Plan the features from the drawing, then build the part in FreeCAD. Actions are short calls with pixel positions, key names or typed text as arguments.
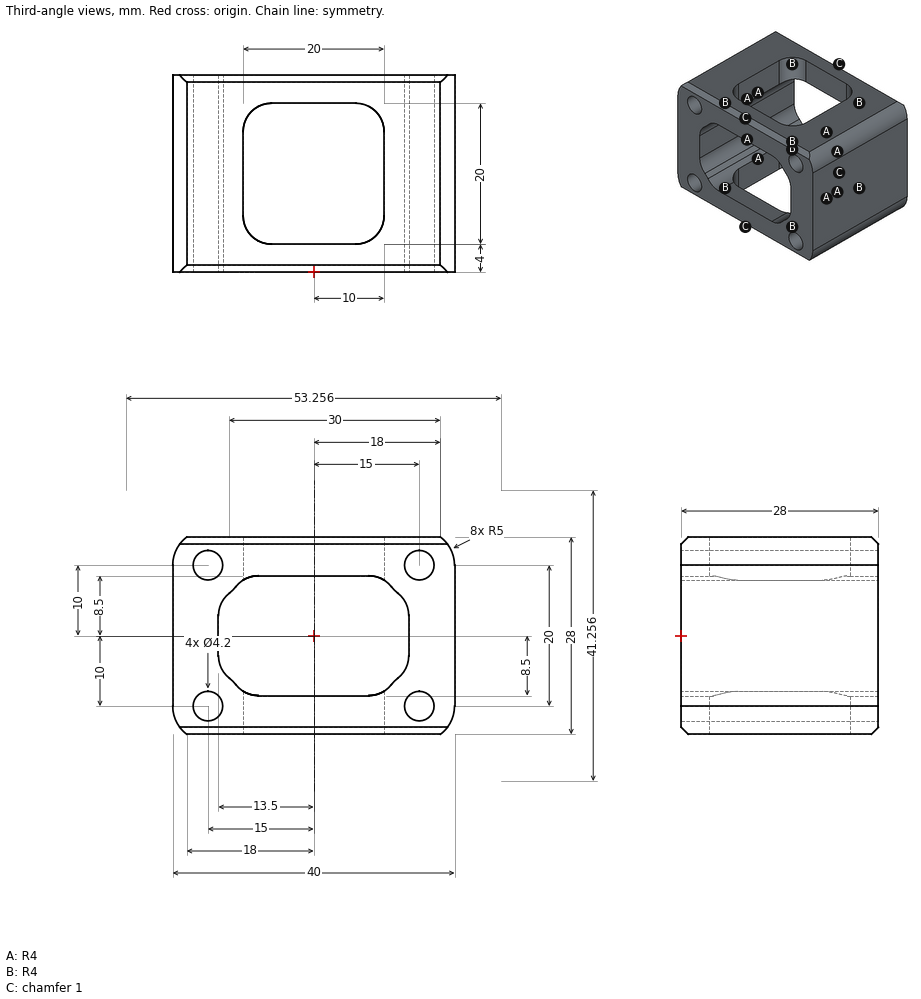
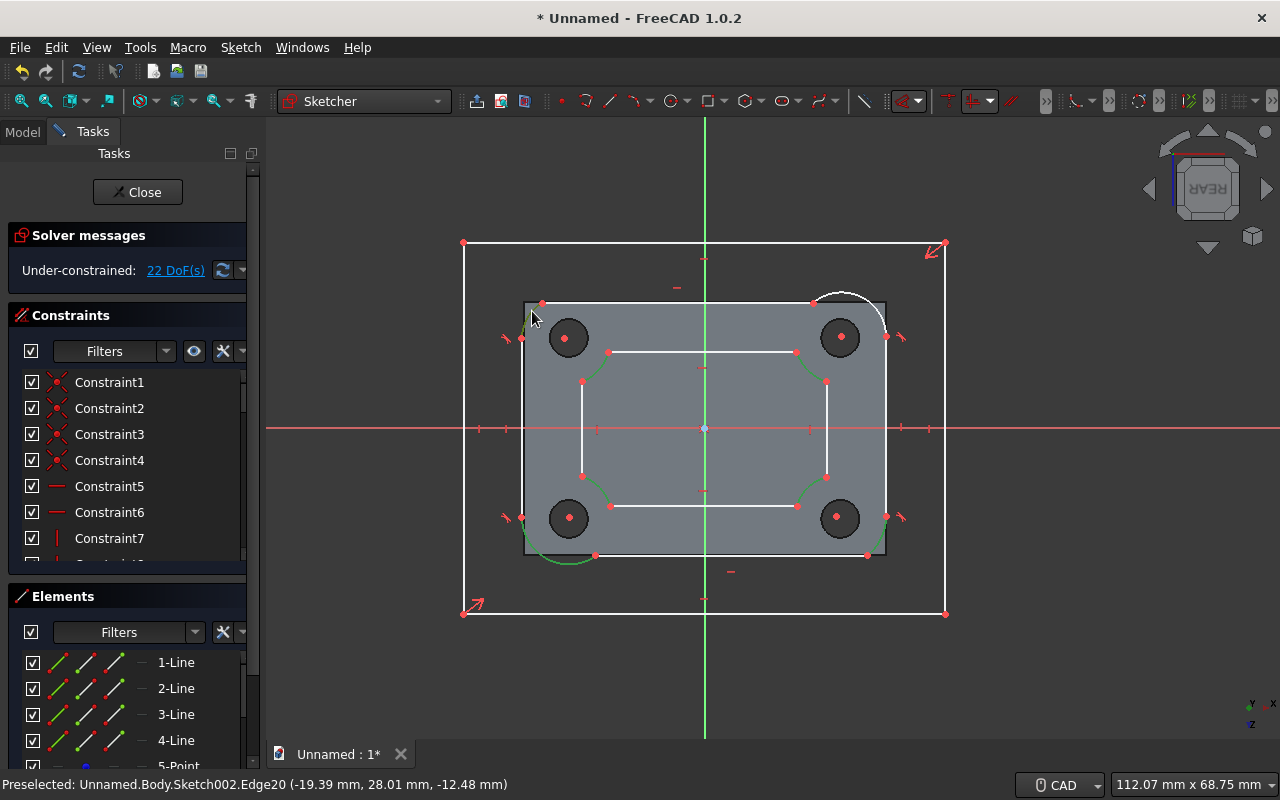
click(876, 309)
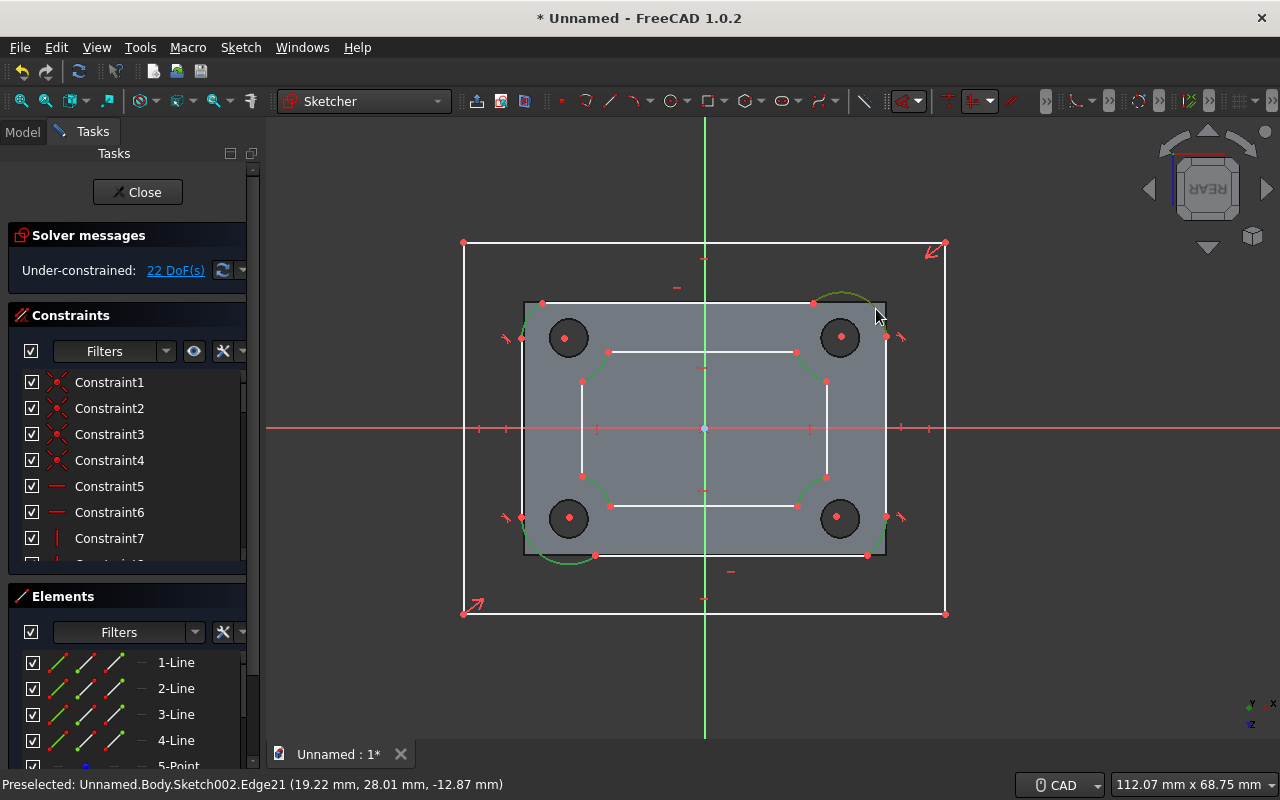
key(e)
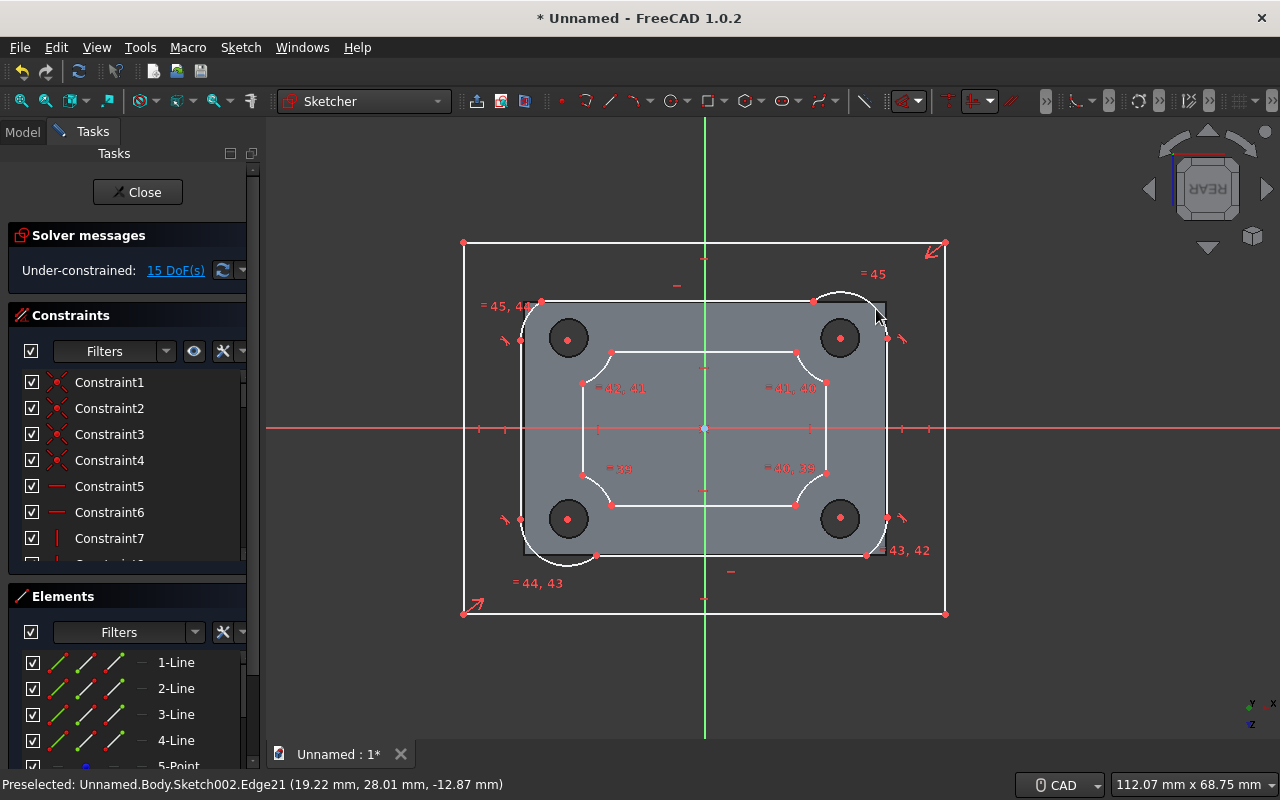
click(567, 519)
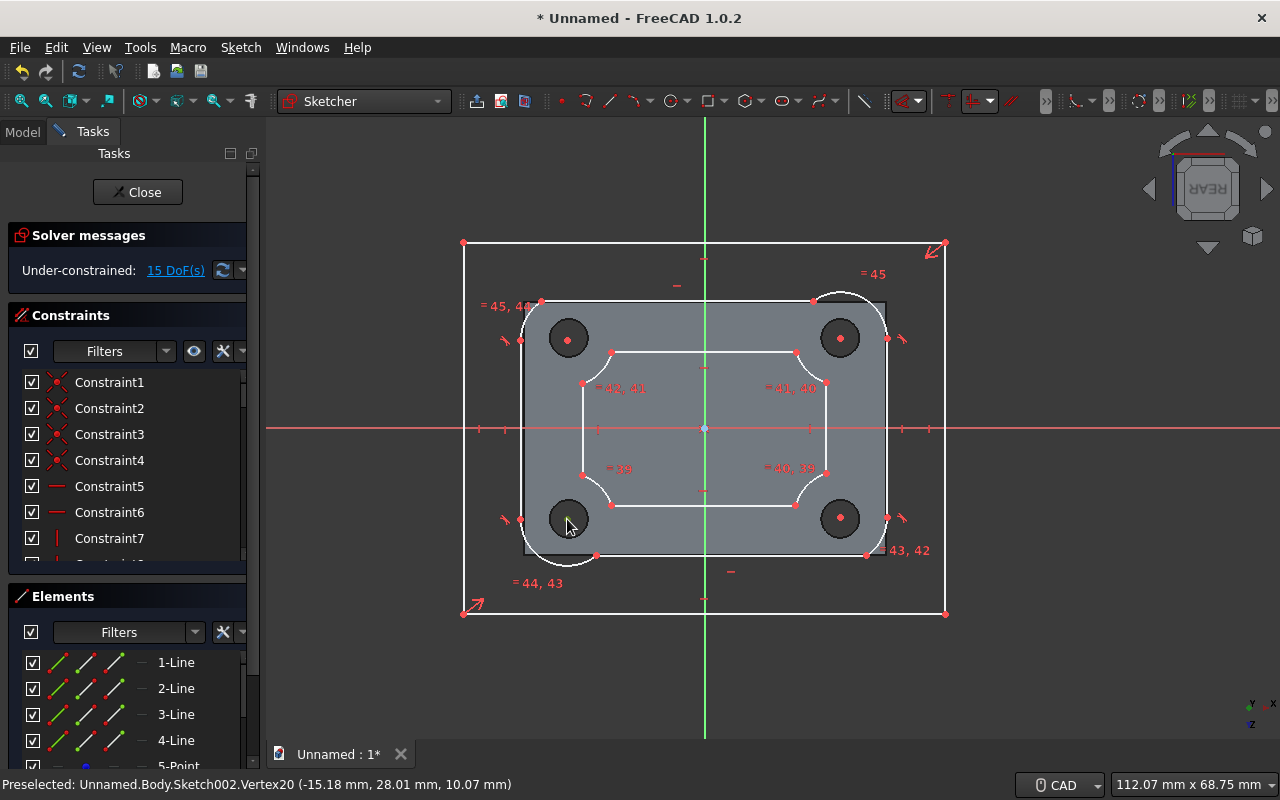
click(841, 518)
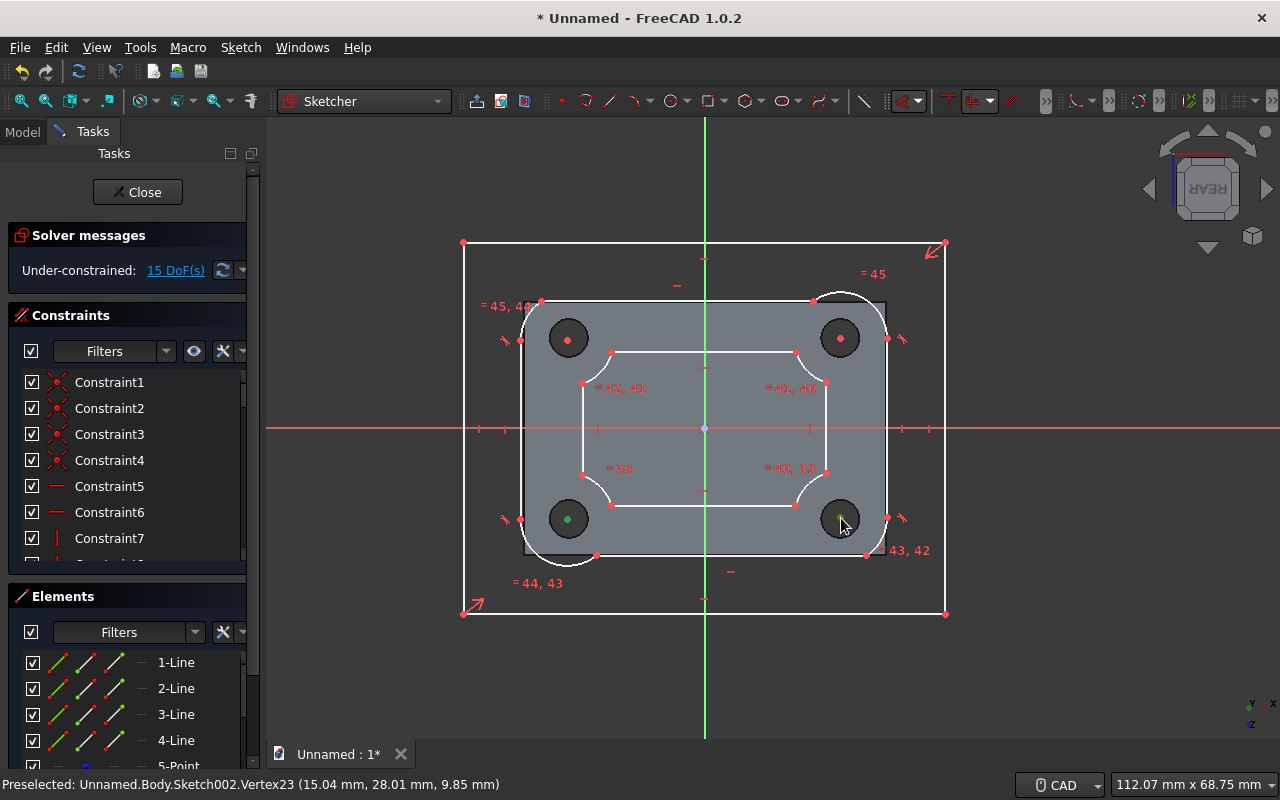
click(705, 671)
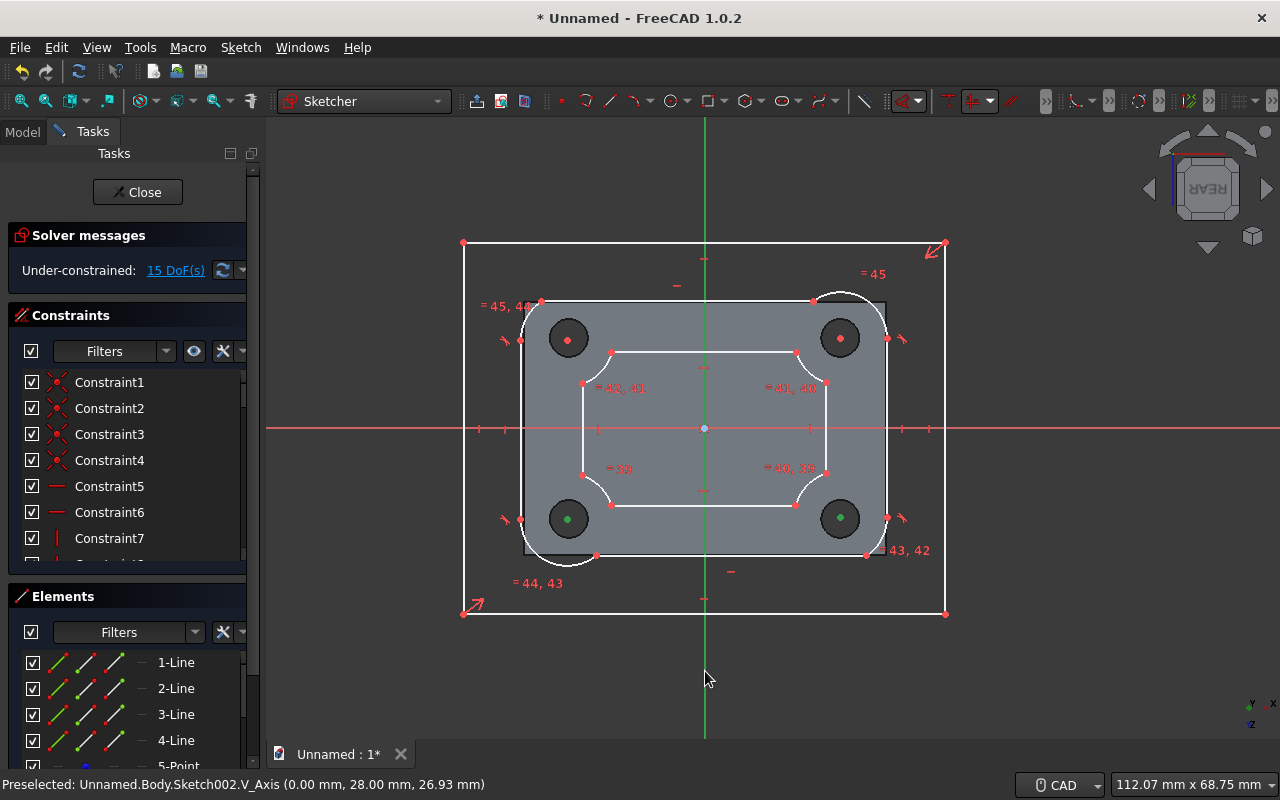
key(s)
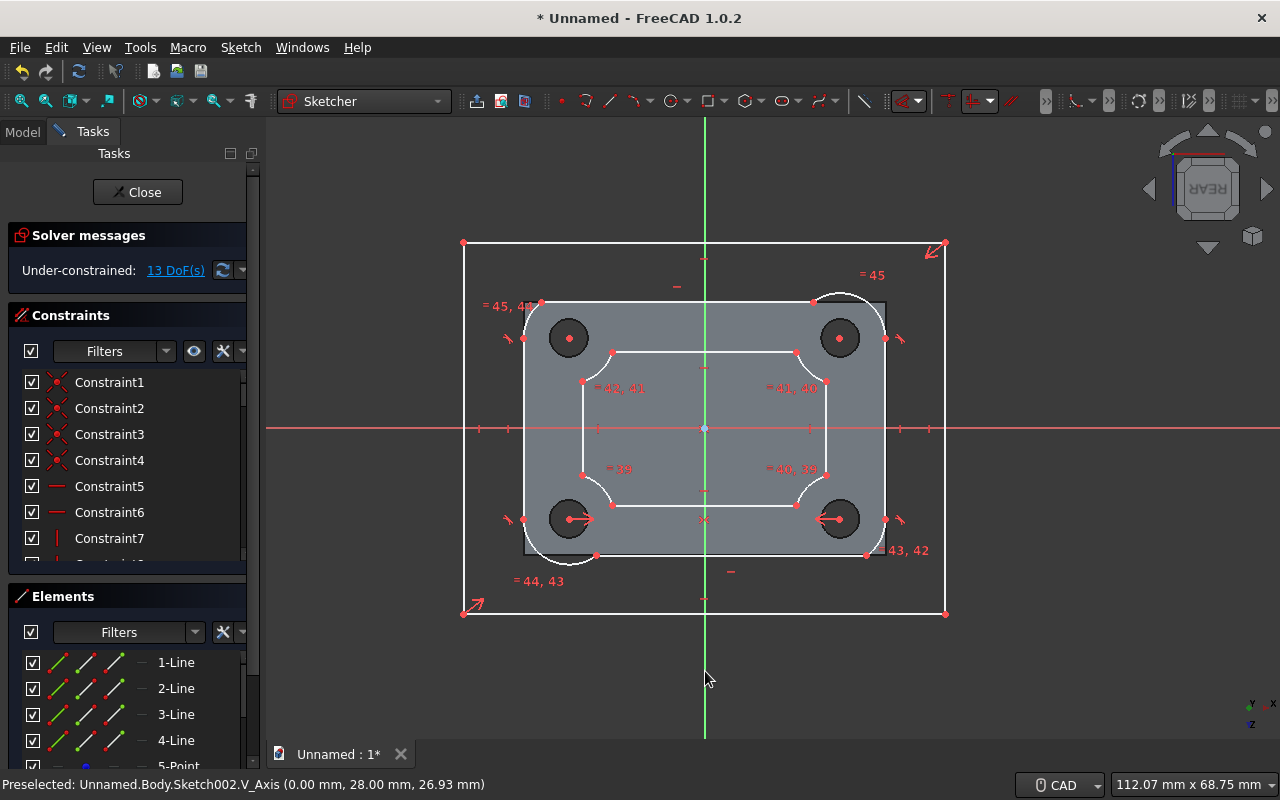
click(583, 382)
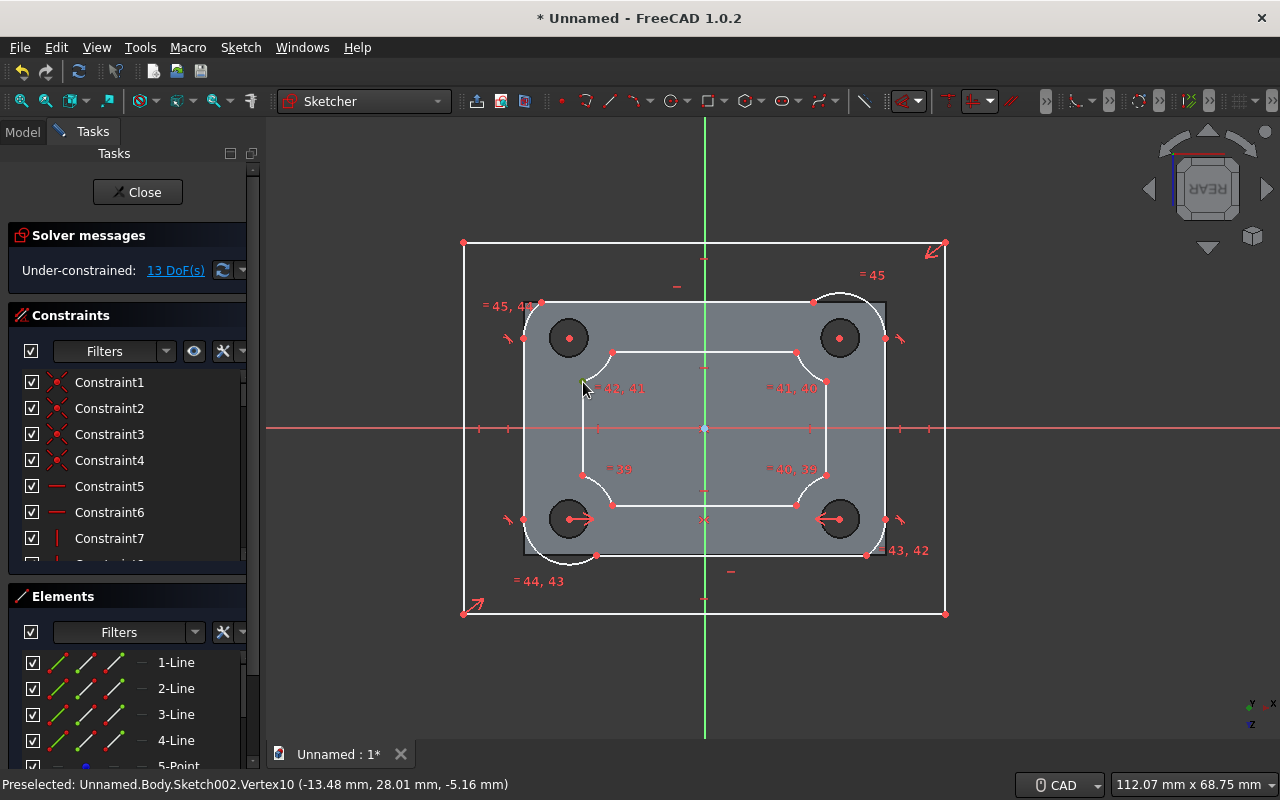
click(826, 382)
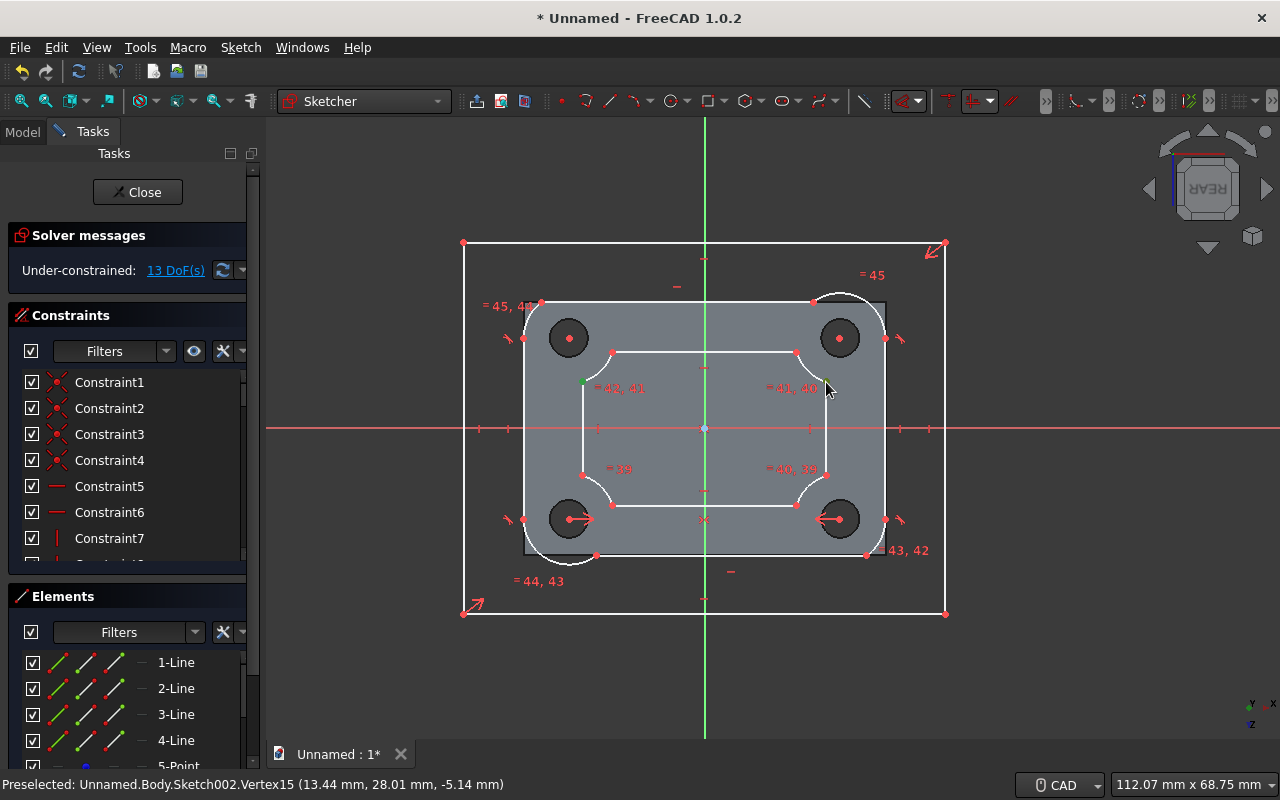
click(705, 671)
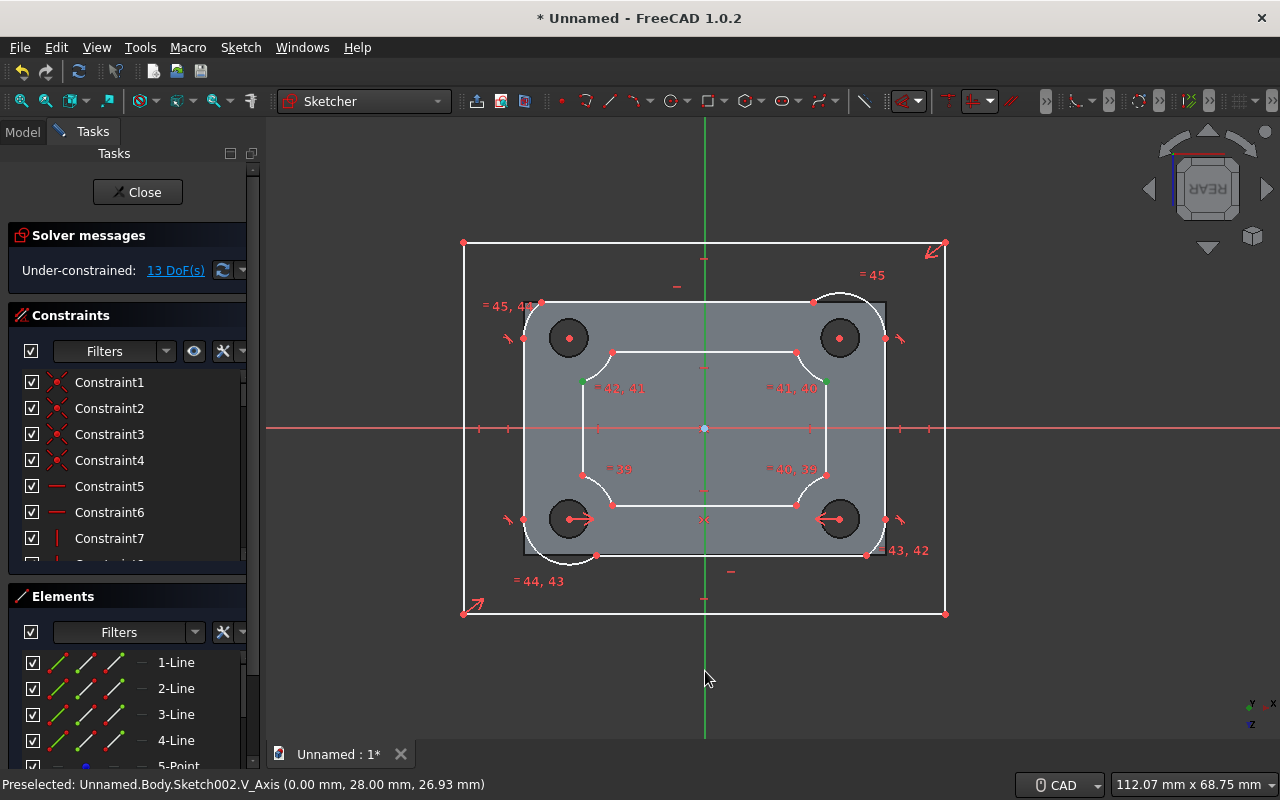
key(s)